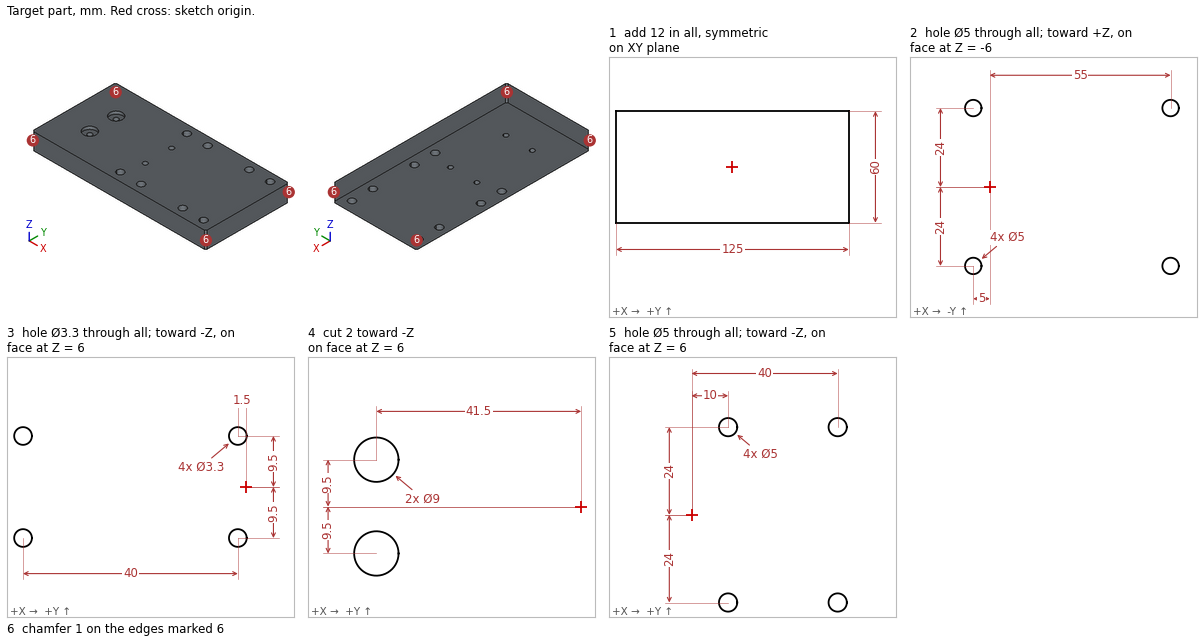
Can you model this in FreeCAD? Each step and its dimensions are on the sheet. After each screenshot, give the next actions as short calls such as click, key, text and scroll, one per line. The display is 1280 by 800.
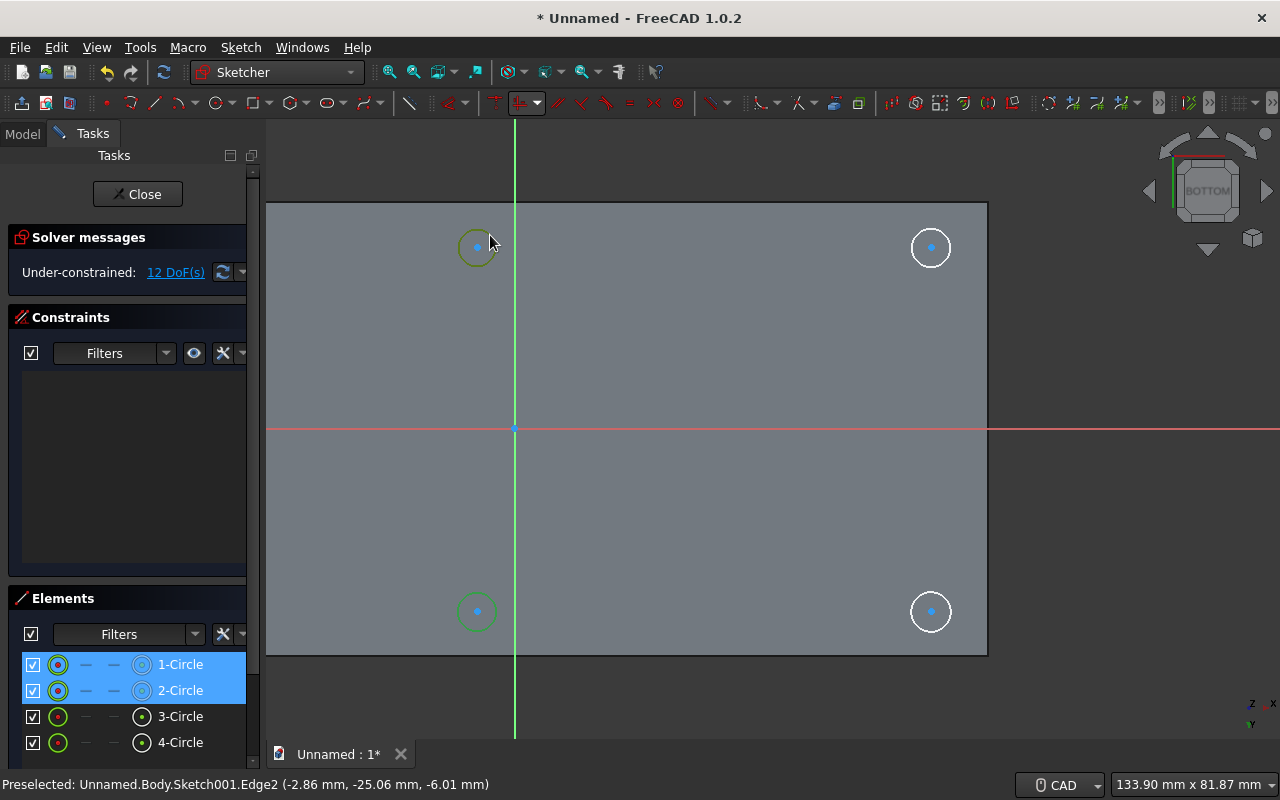
click(944, 234)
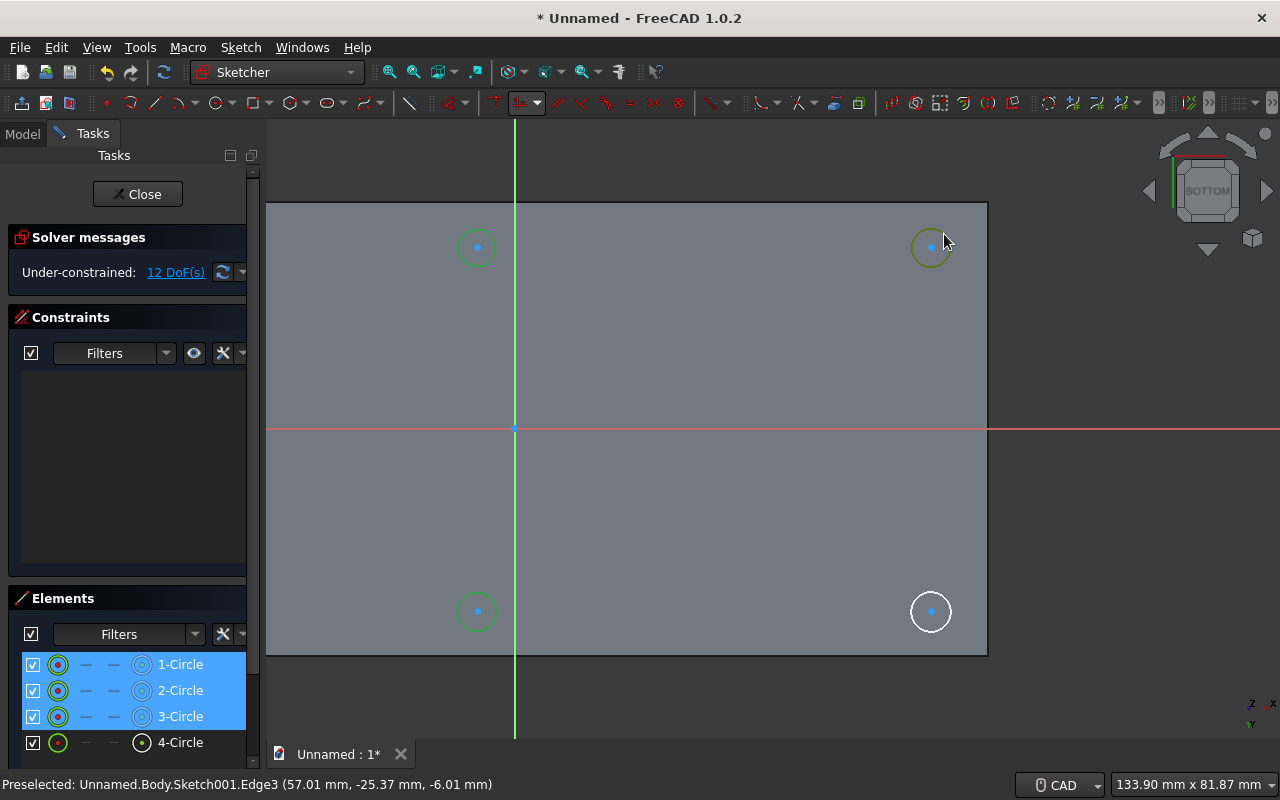
click(945, 598)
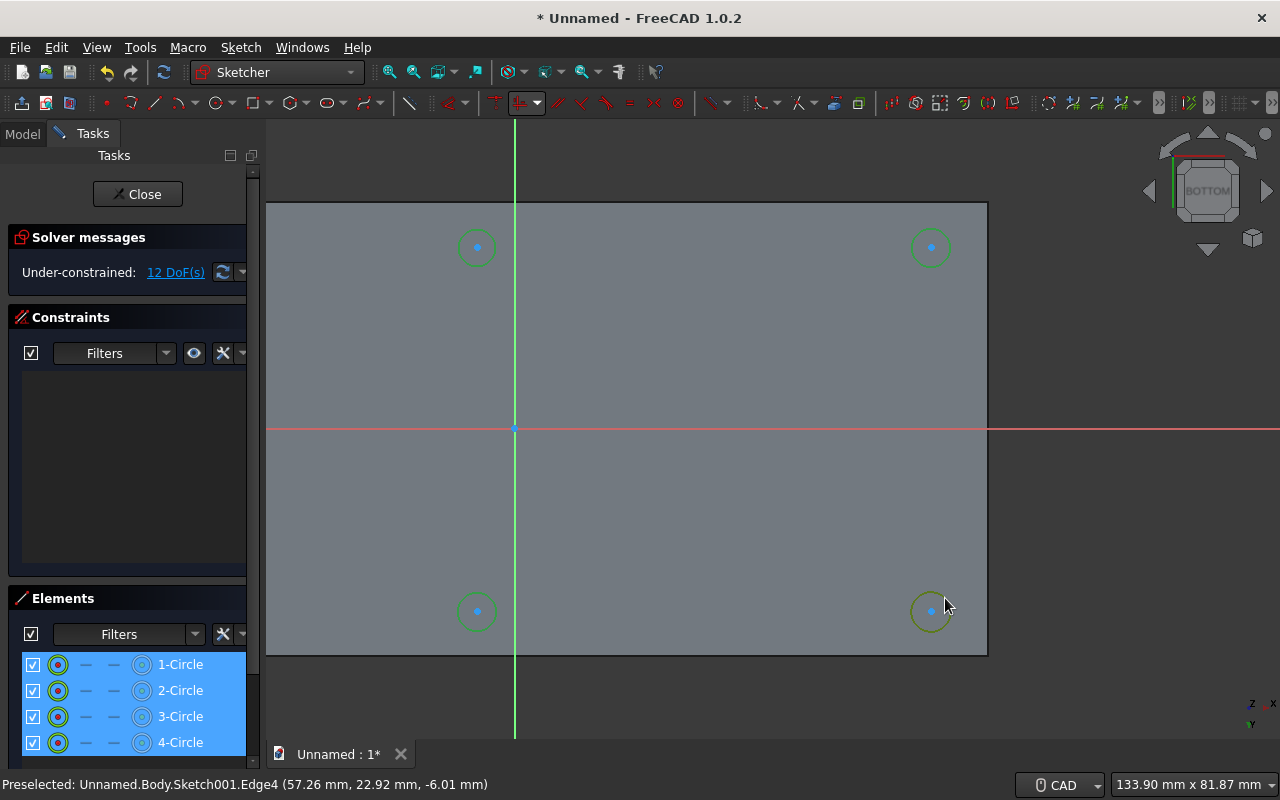
key(e)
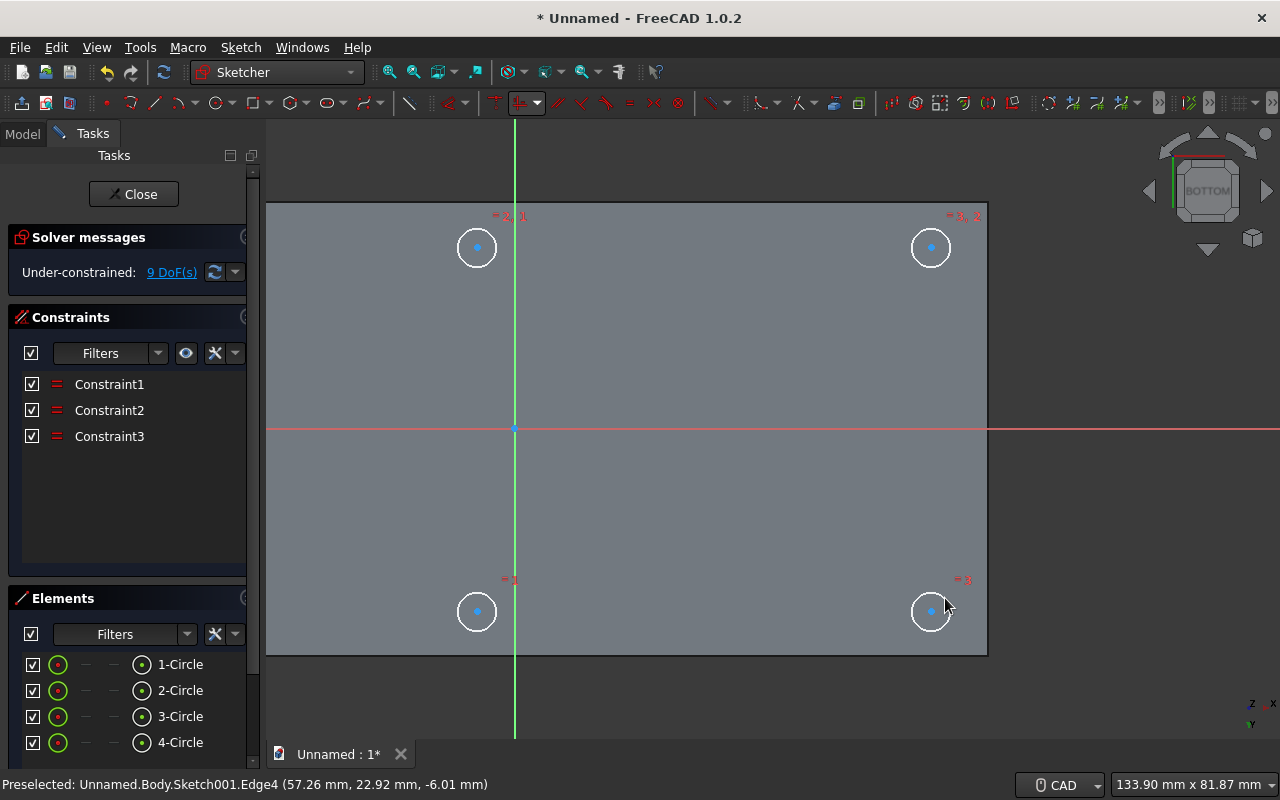
click(477, 612)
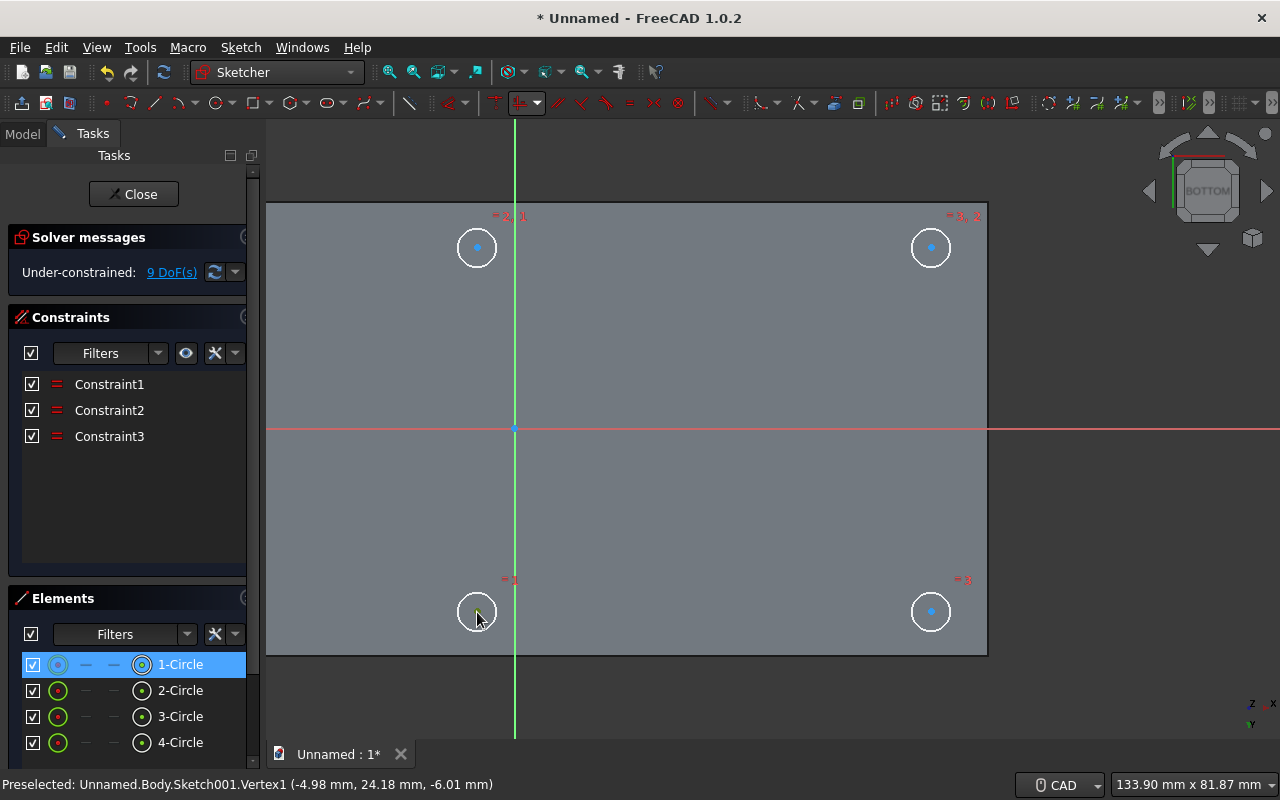
click(477, 248)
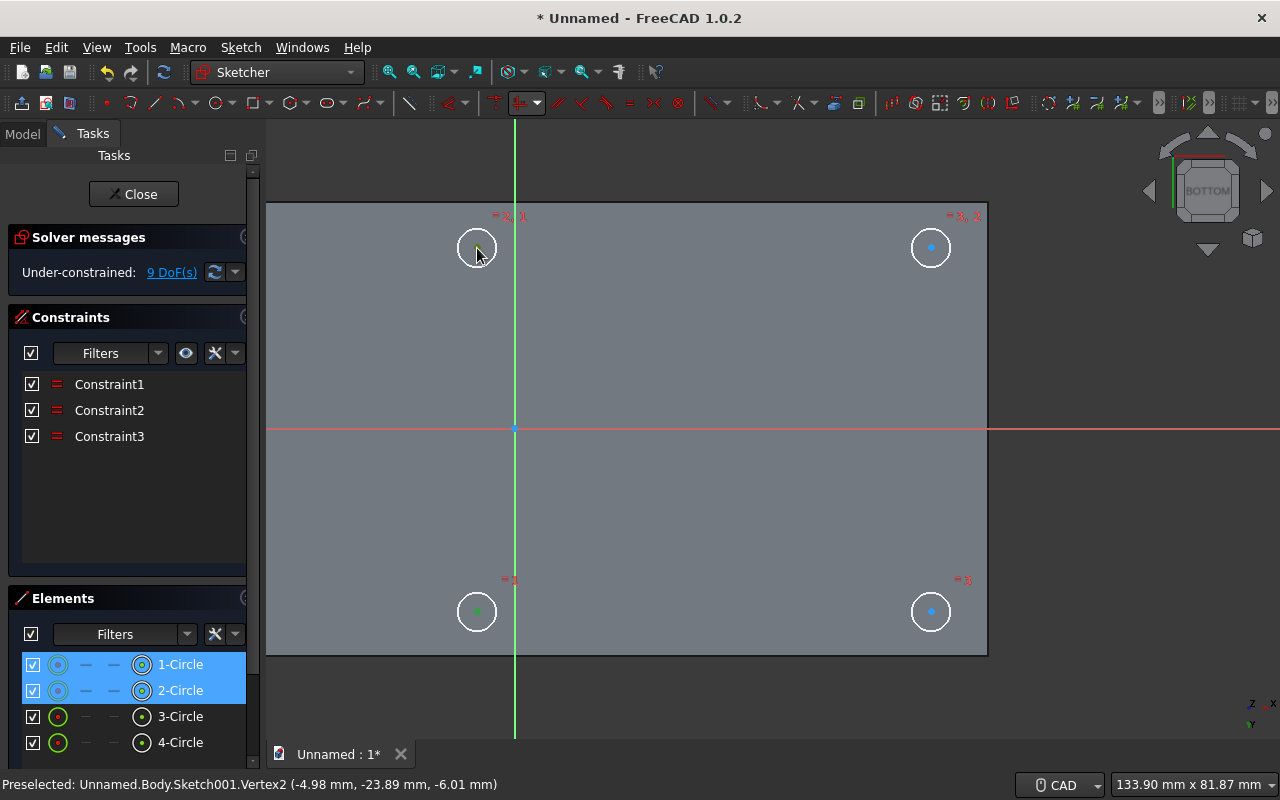
key(v)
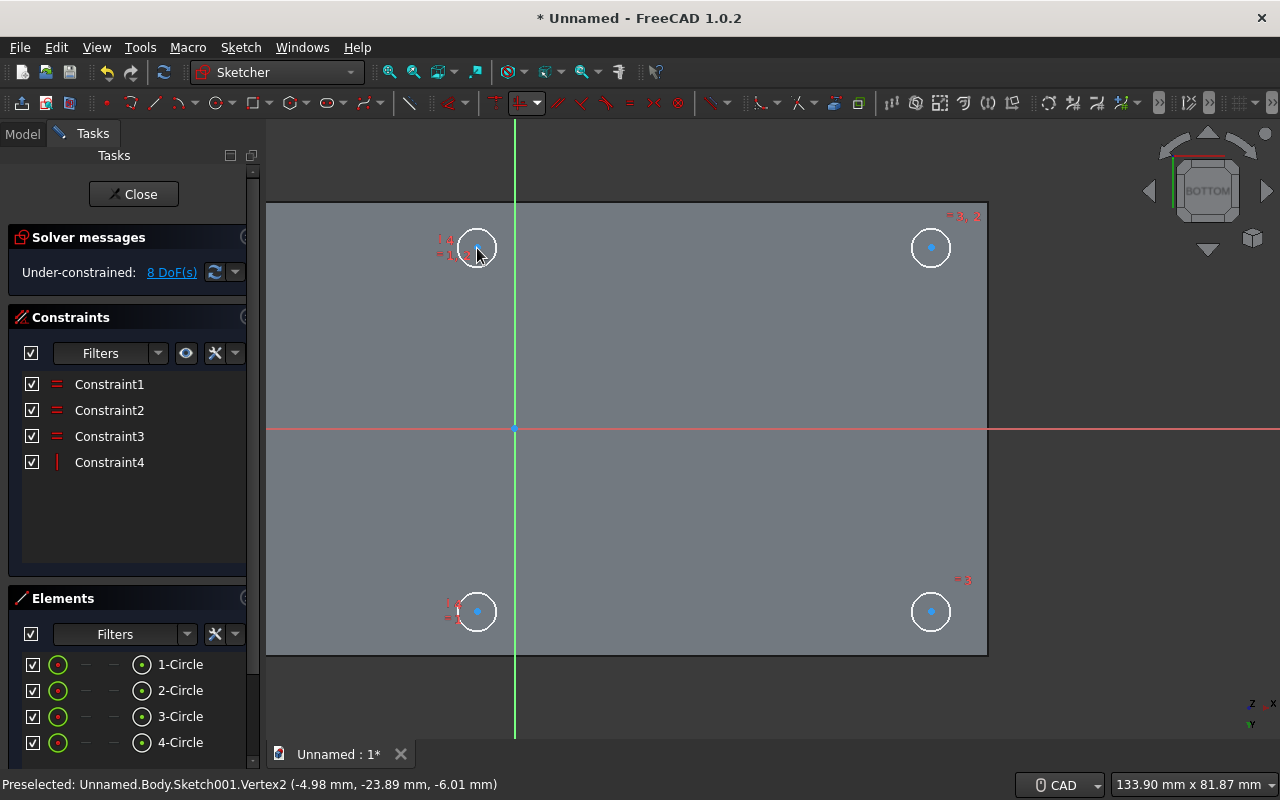
click(477, 248)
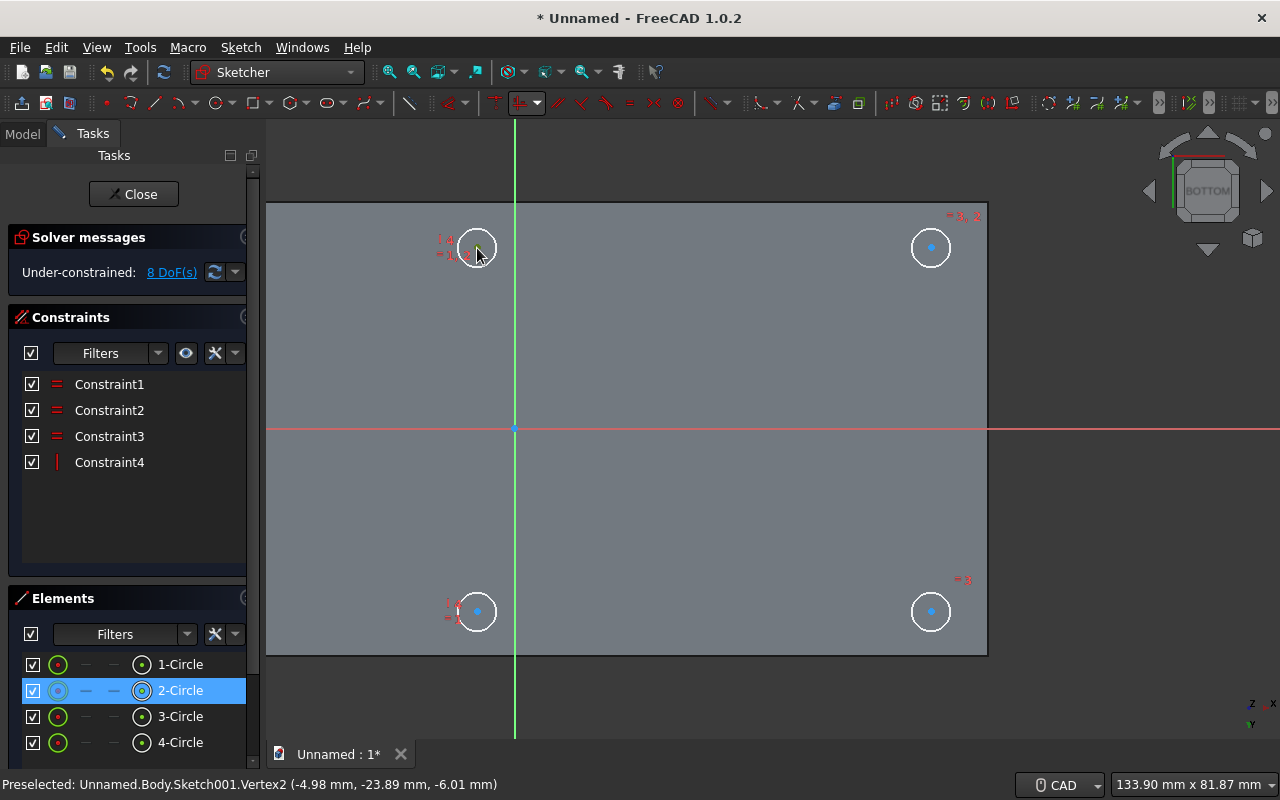
click(931, 248)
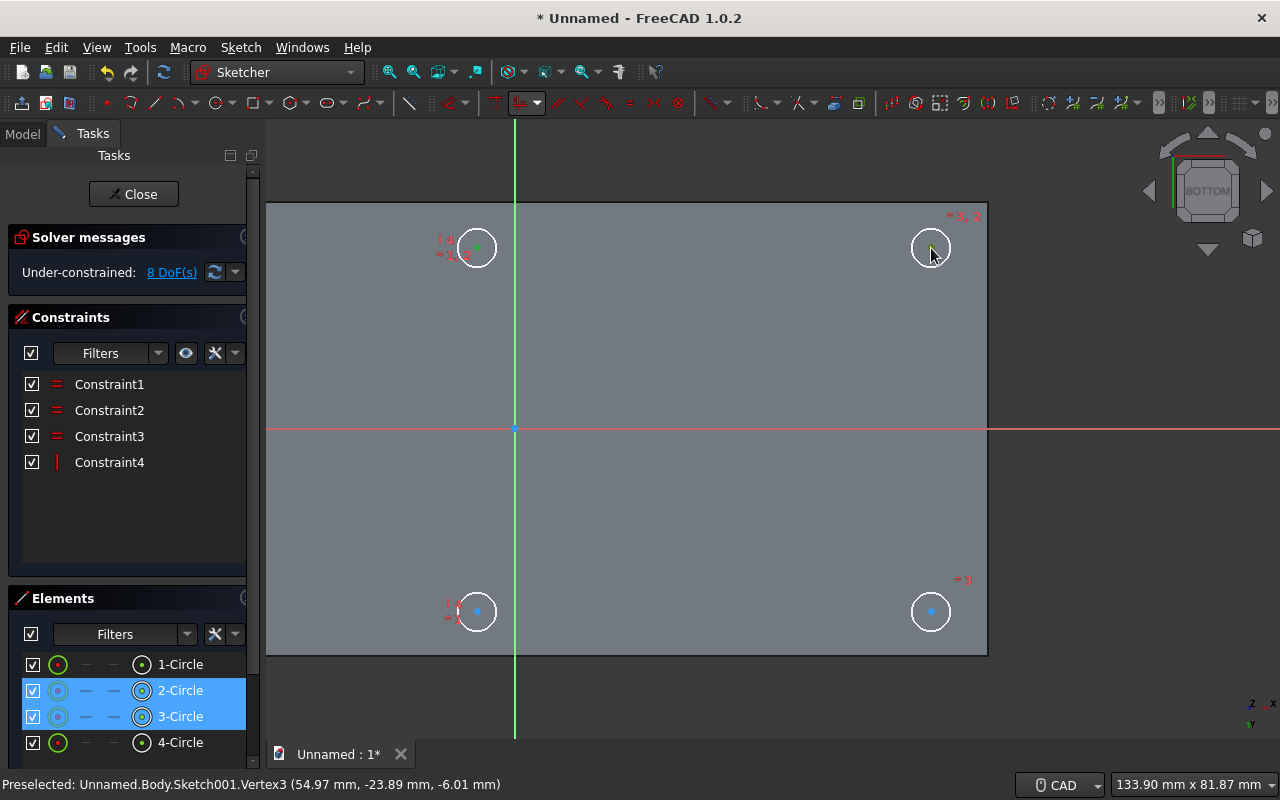
key(h)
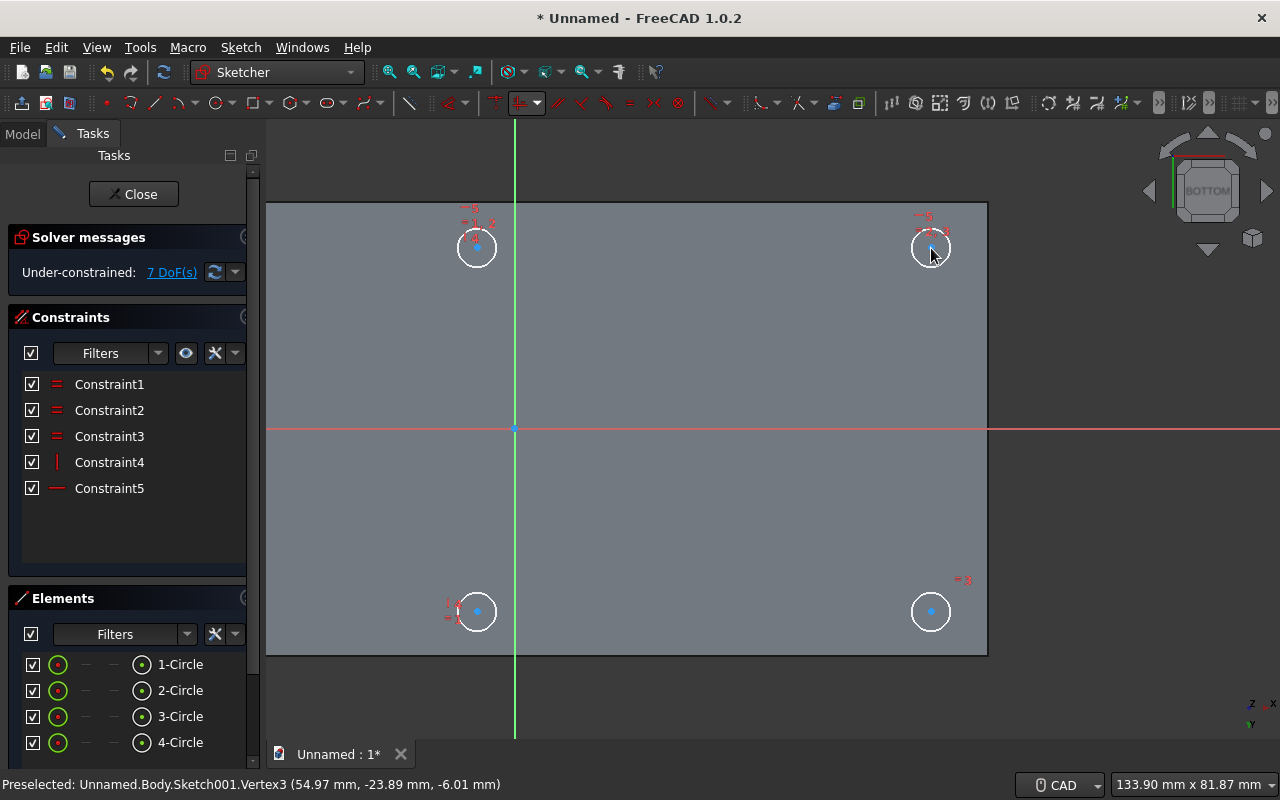
click(931, 248)